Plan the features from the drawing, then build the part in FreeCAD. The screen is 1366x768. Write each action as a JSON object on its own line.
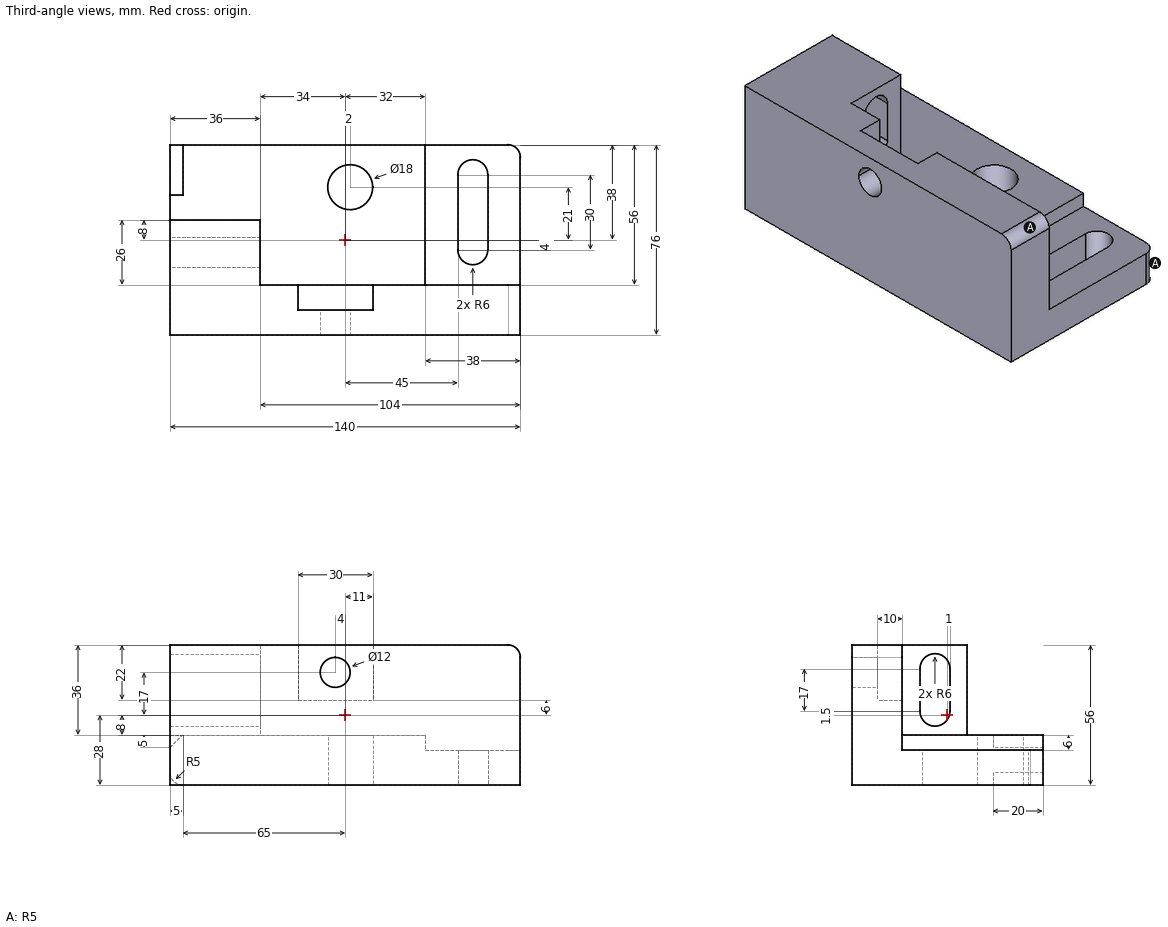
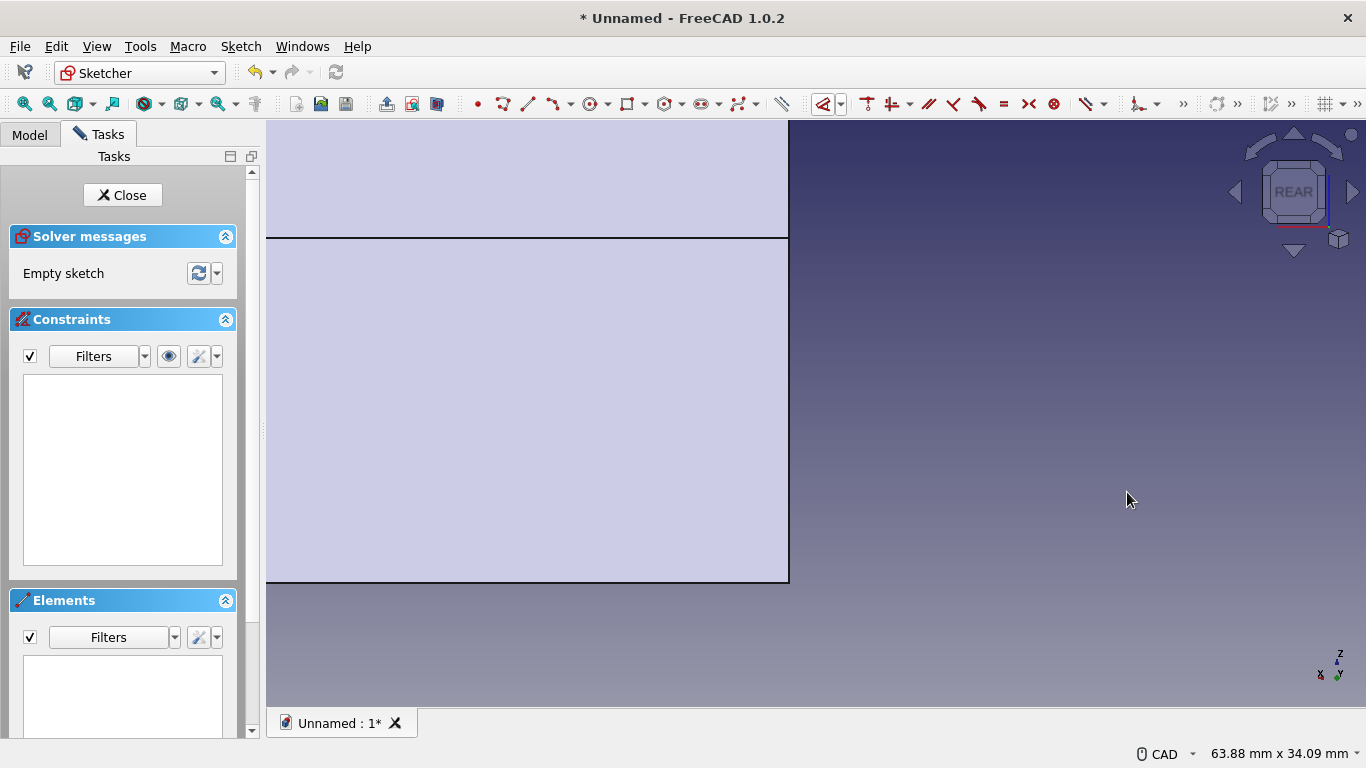
{"action": "left_click", "coordinate": [503, 104]}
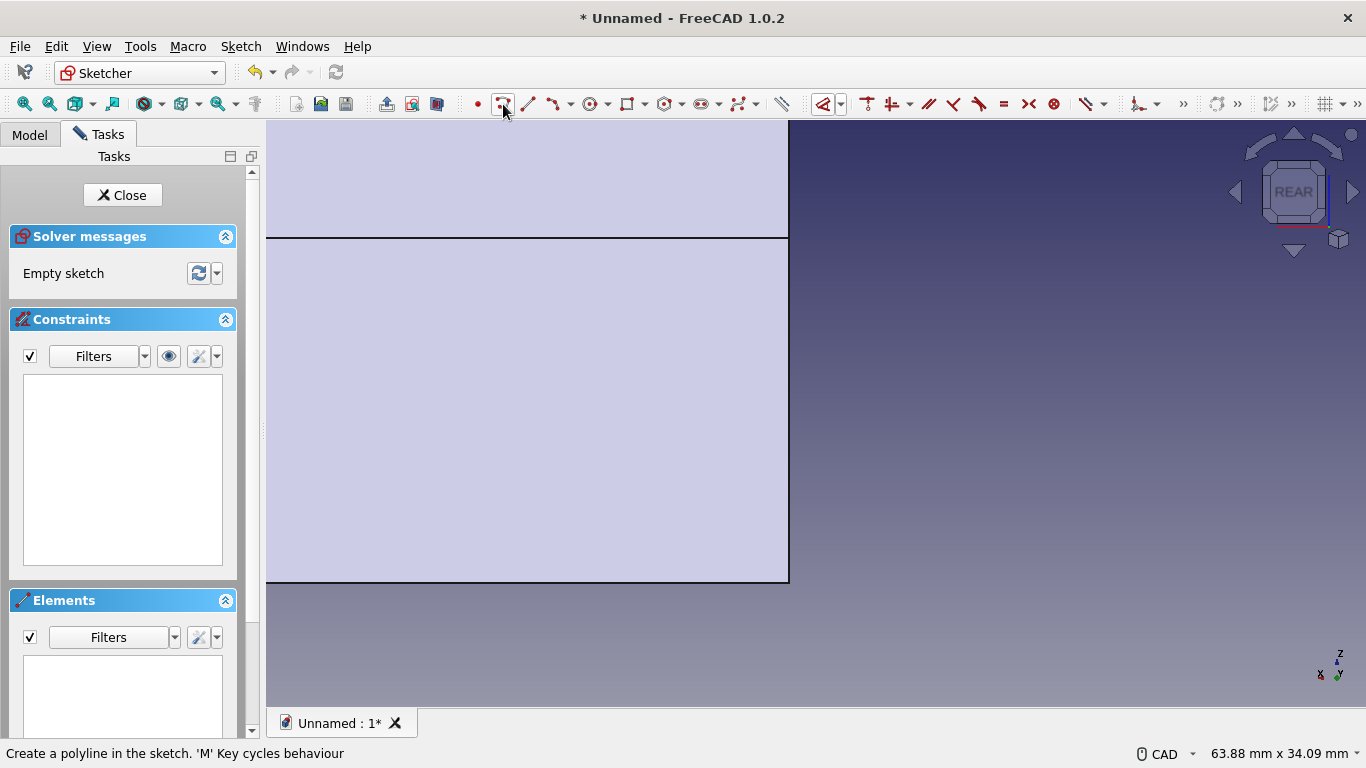
{"action": "left_click", "coordinate": [703, 238]}
{"action": "left_click", "coordinate": [789, 325]}
{"action": "left_click", "coordinate": [789, 238]}
{"action": "left_click", "coordinate": [703, 239]}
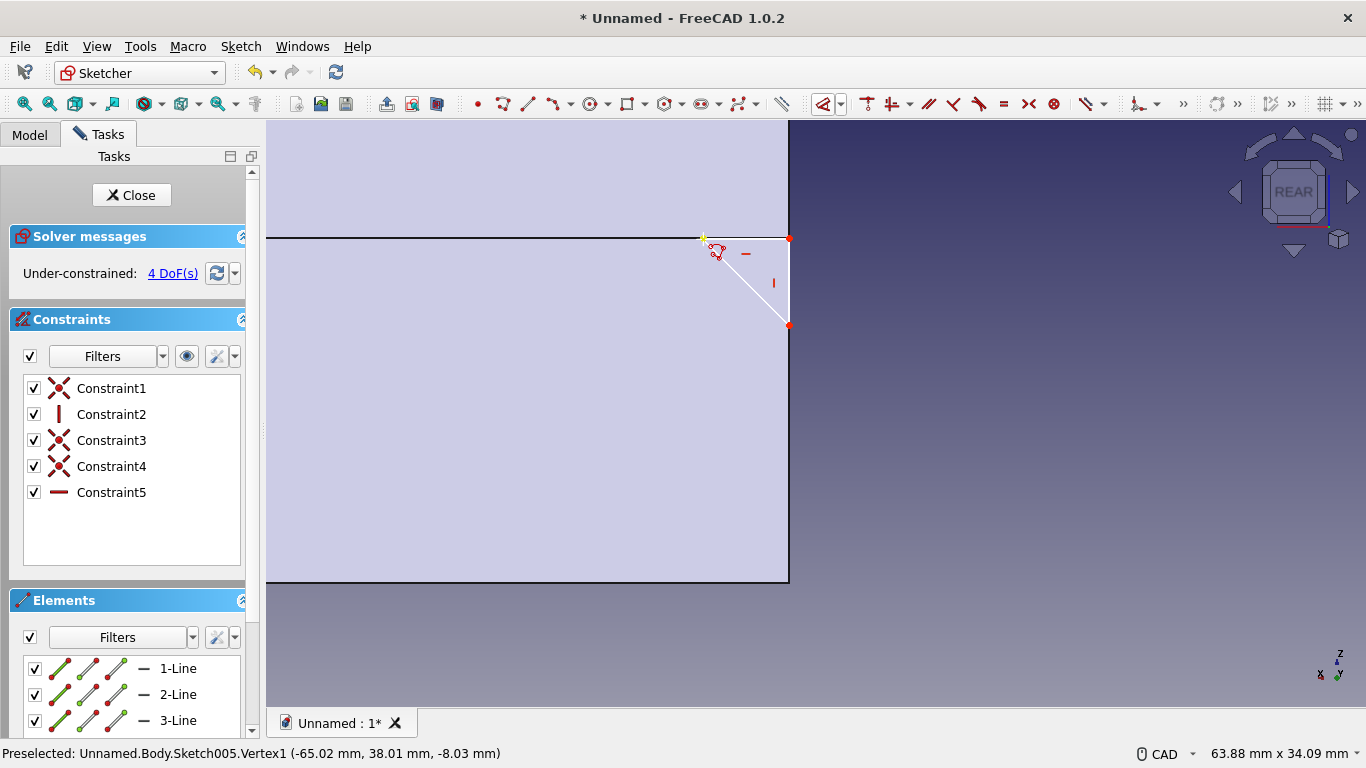
{"action": "left_click", "coordinate": [703, 583]}
{"action": "left_click", "coordinate": [789, 583]}
{"action": "left_click", "coordinate": [789, 497]}
{"action": "right_click", "coordinate": [789, 497]}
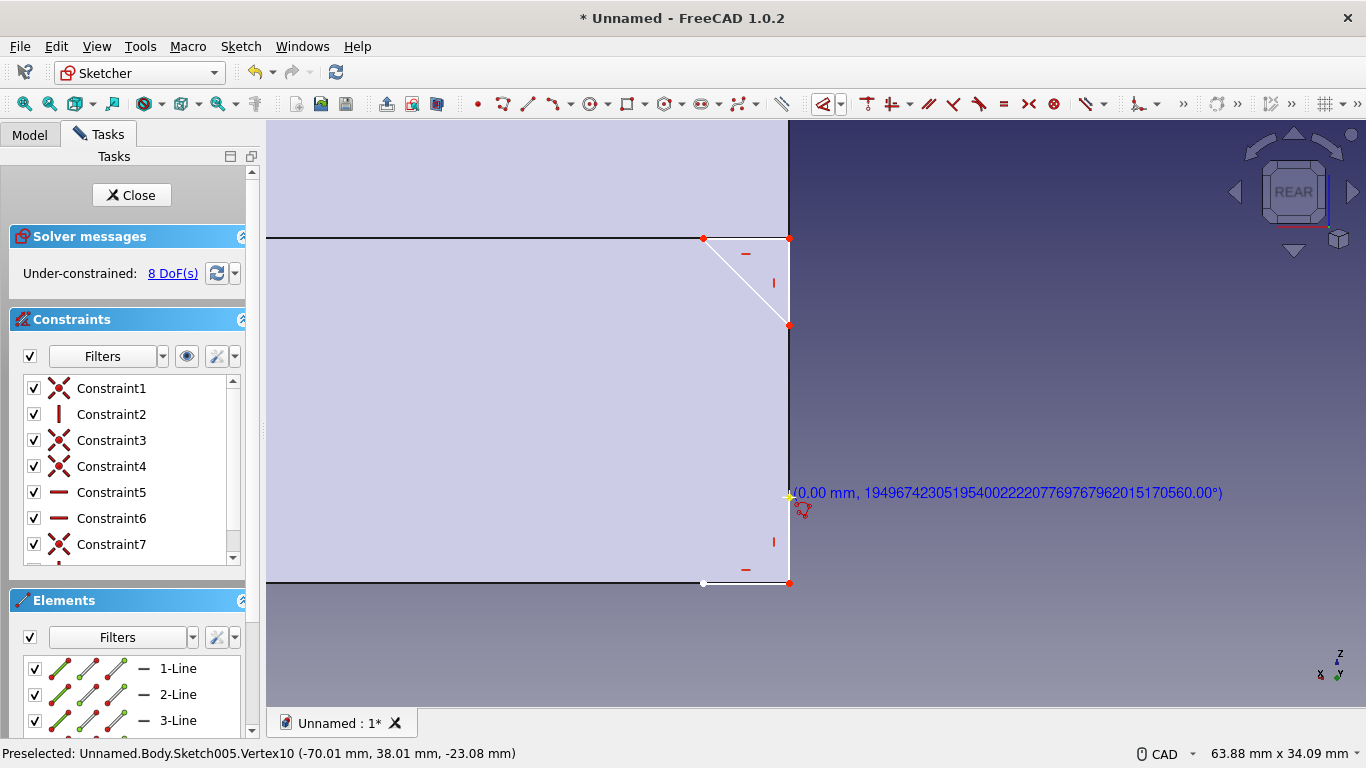
{"action": "left_click", "coordinate": [552, 104]}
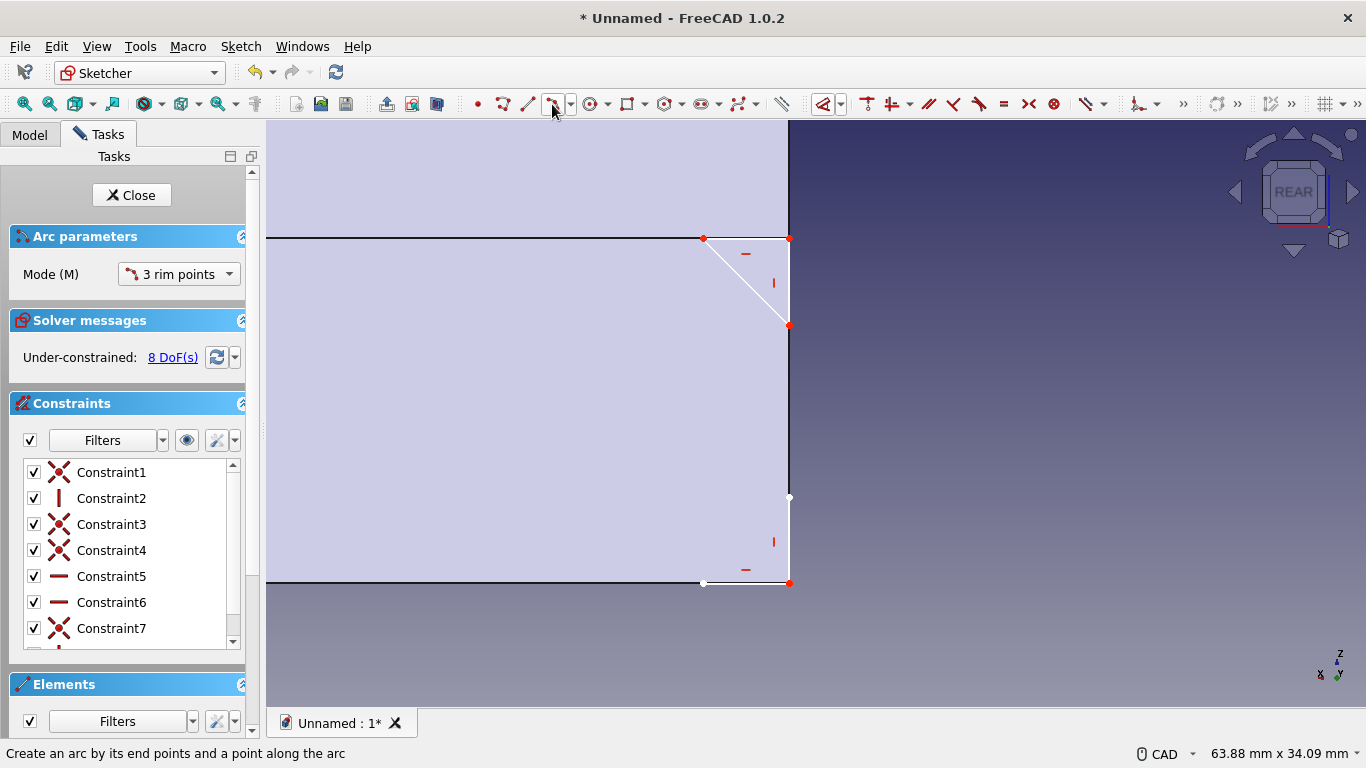
{"action": "left_click", "coordinate": [789, 498]}
{"action": "left_click", "coordinate": [703, 584]}
{"action": "left_click", "coordinate": [764, 558]}
{"action": "key", "text": "Escape"}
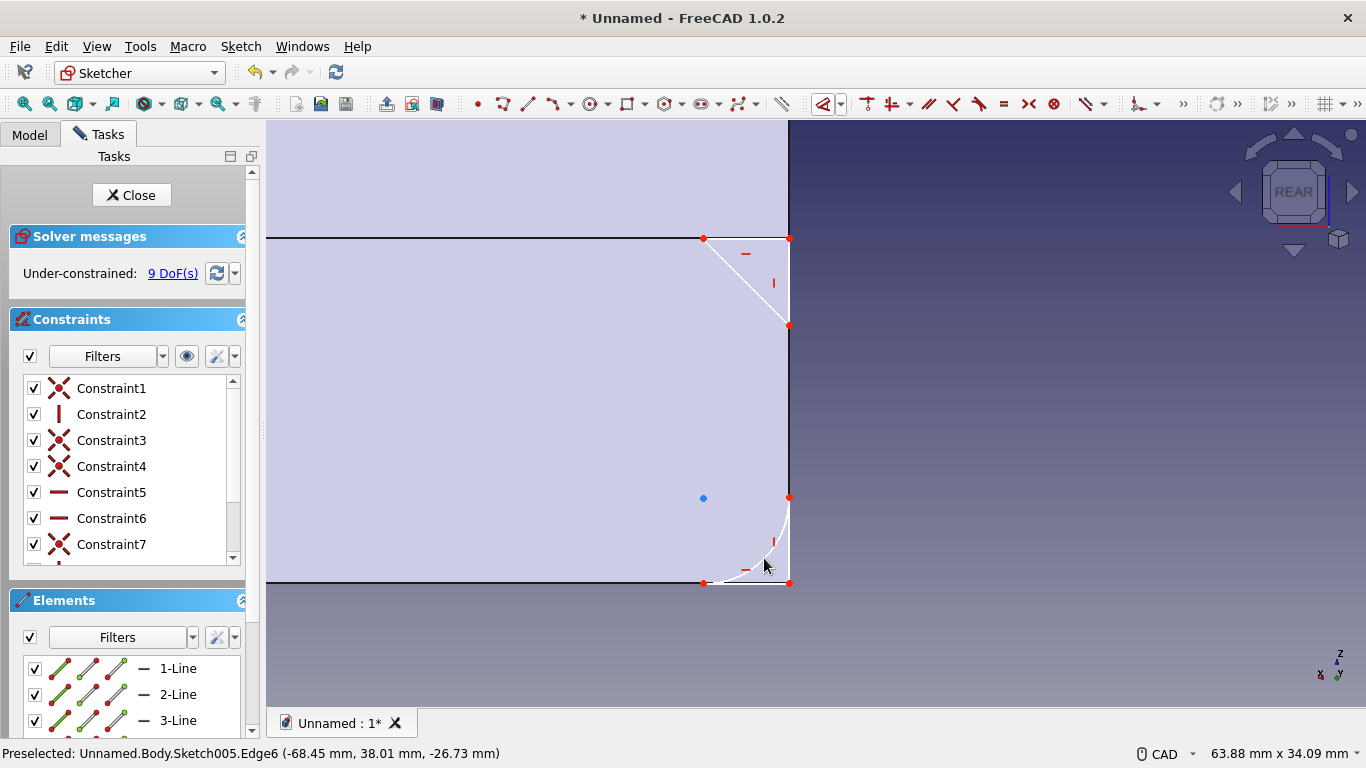
{"action": "left_click", "coordinate": [763, 584]}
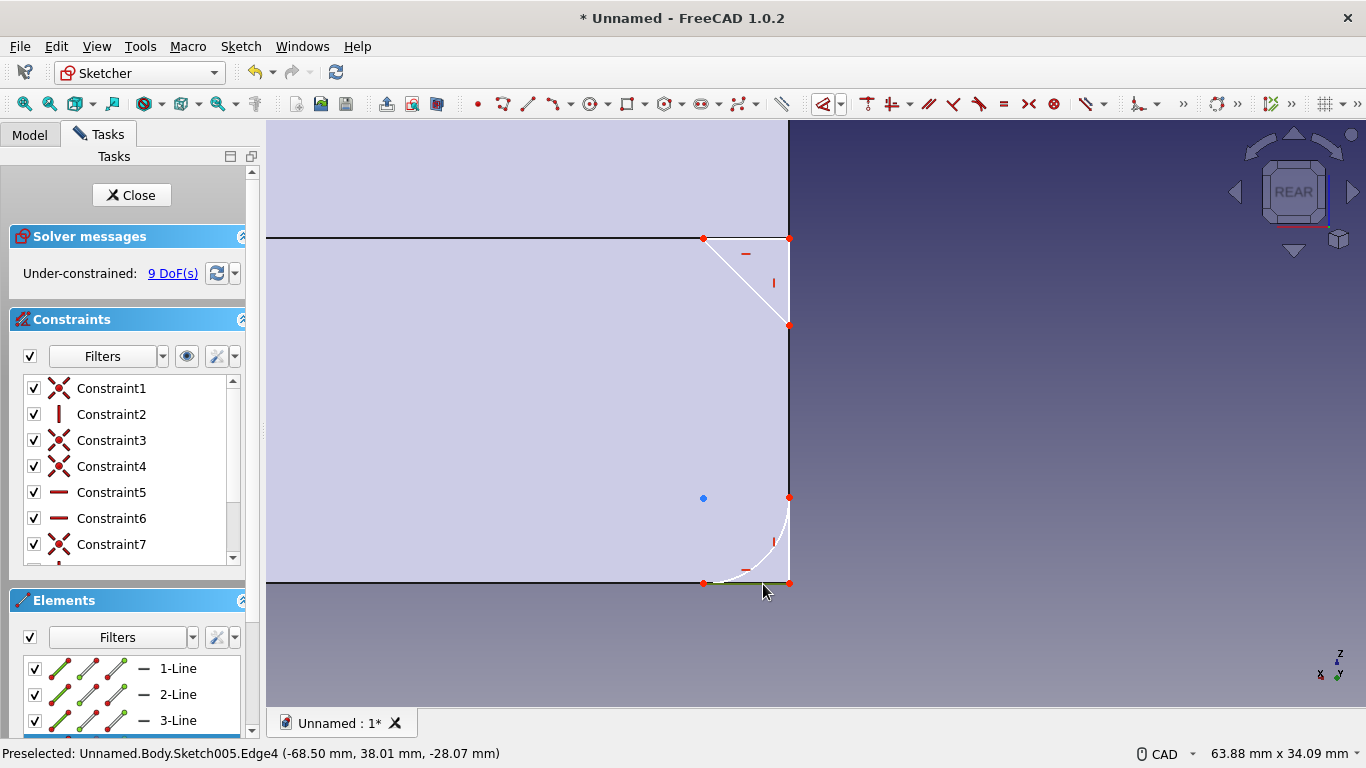
{"action": "scroll", "coordinate": [742, 575], "scroll_direction": "up", "scroll_amount": 3}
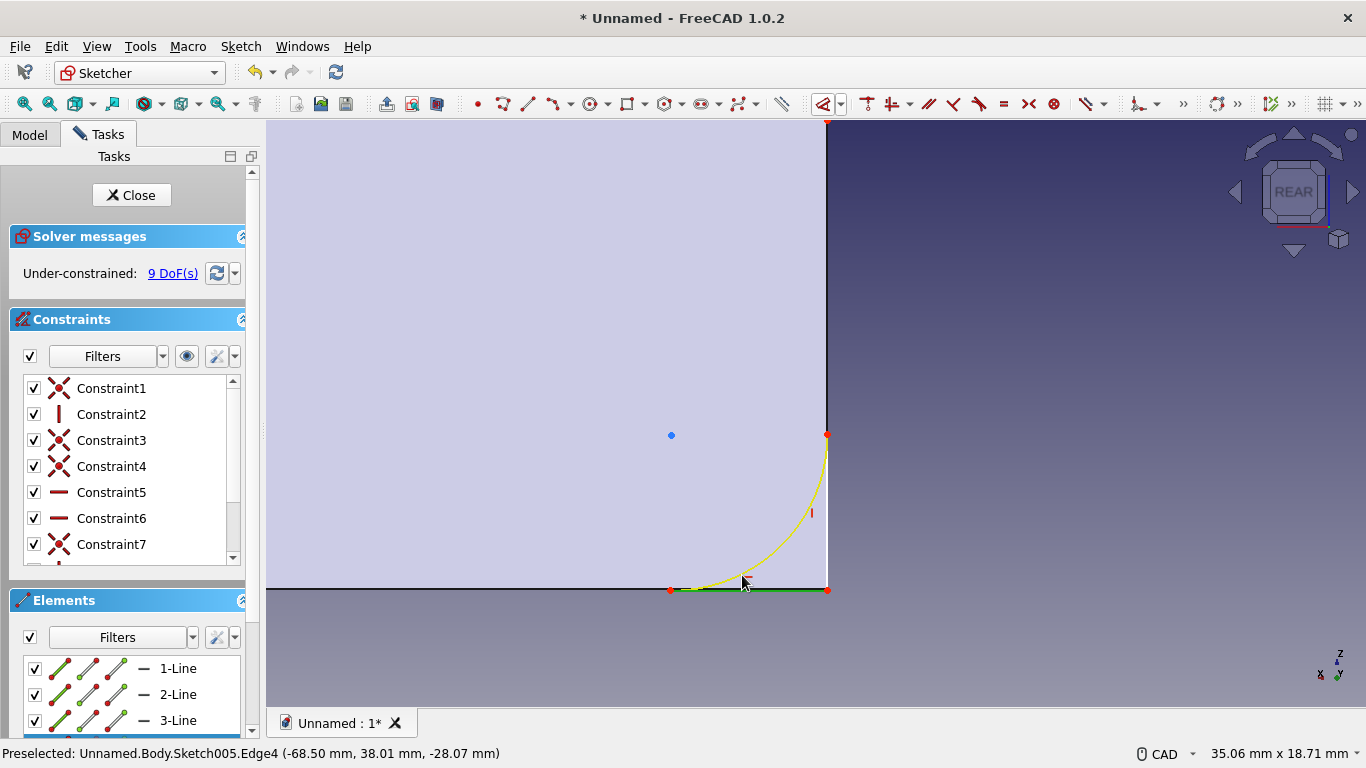
{"action": "left_click", "coordinate": [742, 574]}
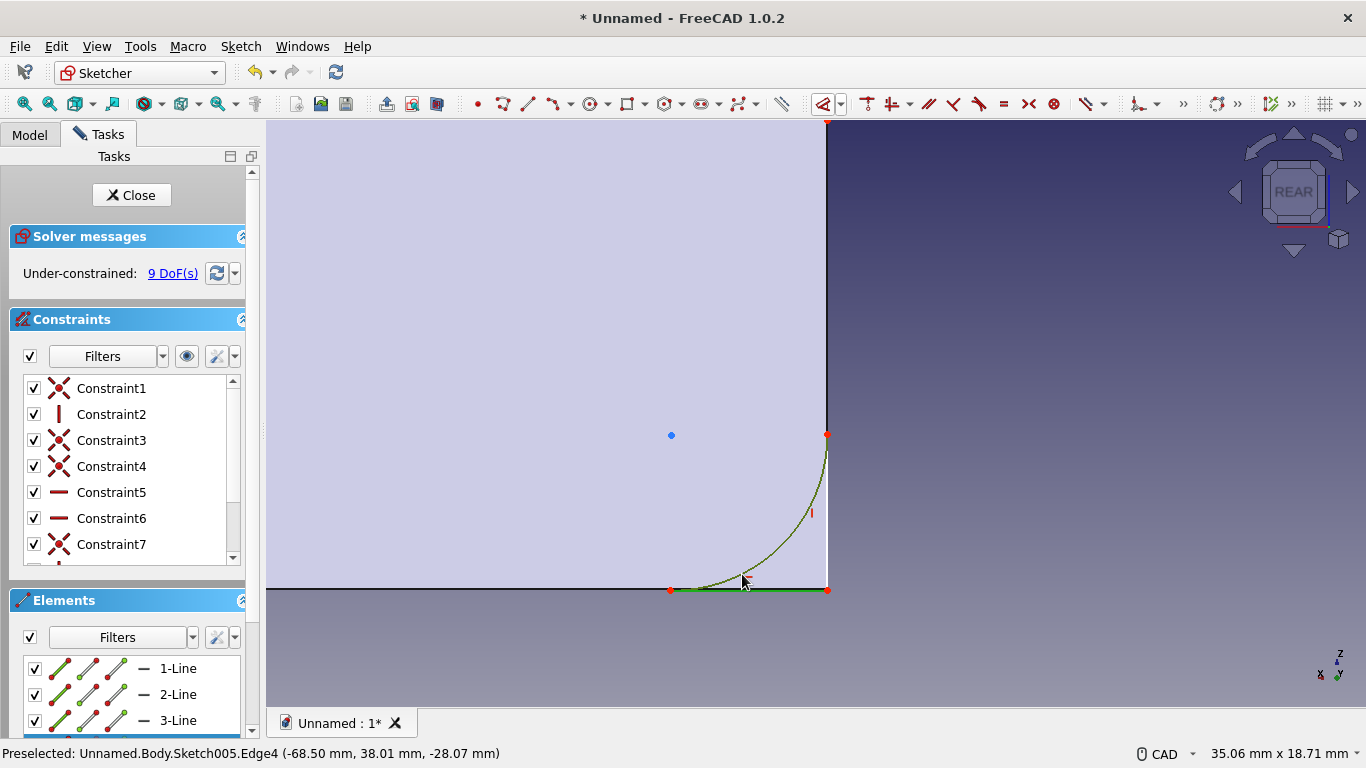
{"action": "left_click", "coordinate": [979, 104]}